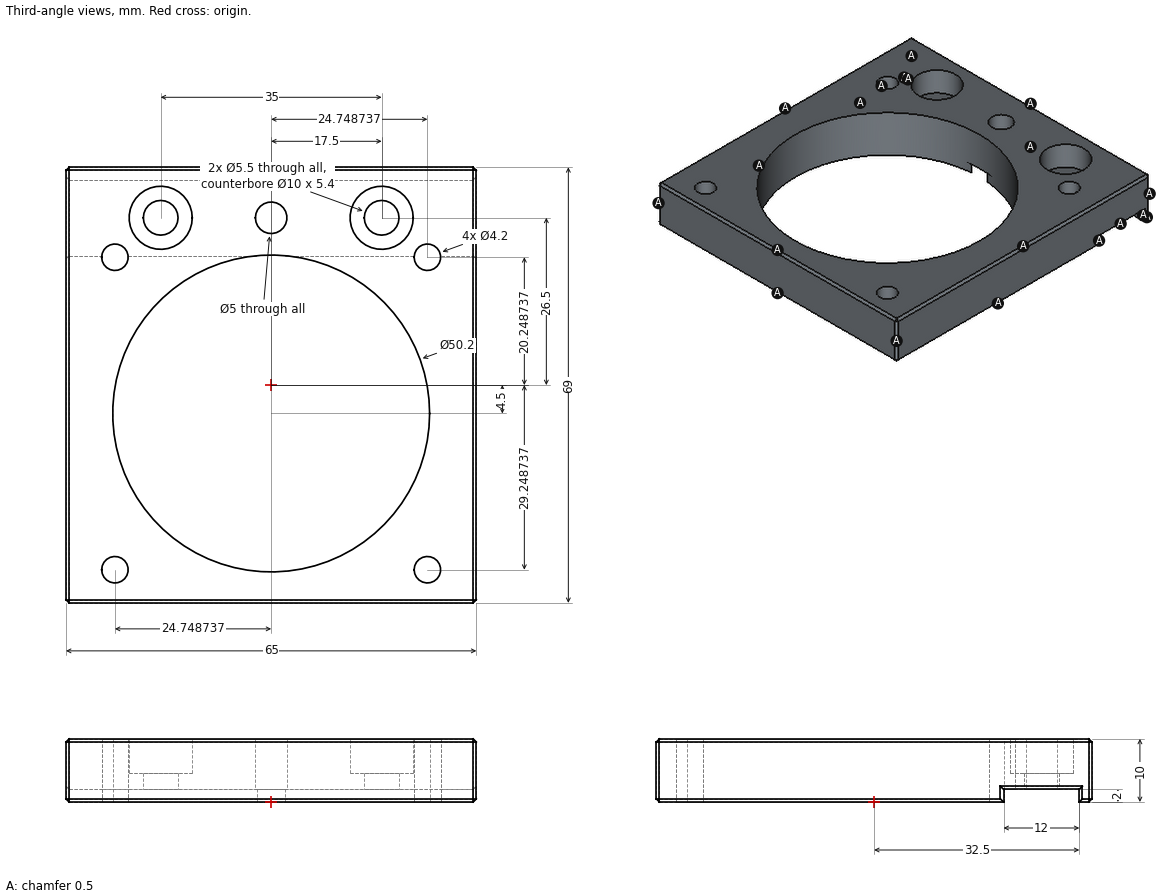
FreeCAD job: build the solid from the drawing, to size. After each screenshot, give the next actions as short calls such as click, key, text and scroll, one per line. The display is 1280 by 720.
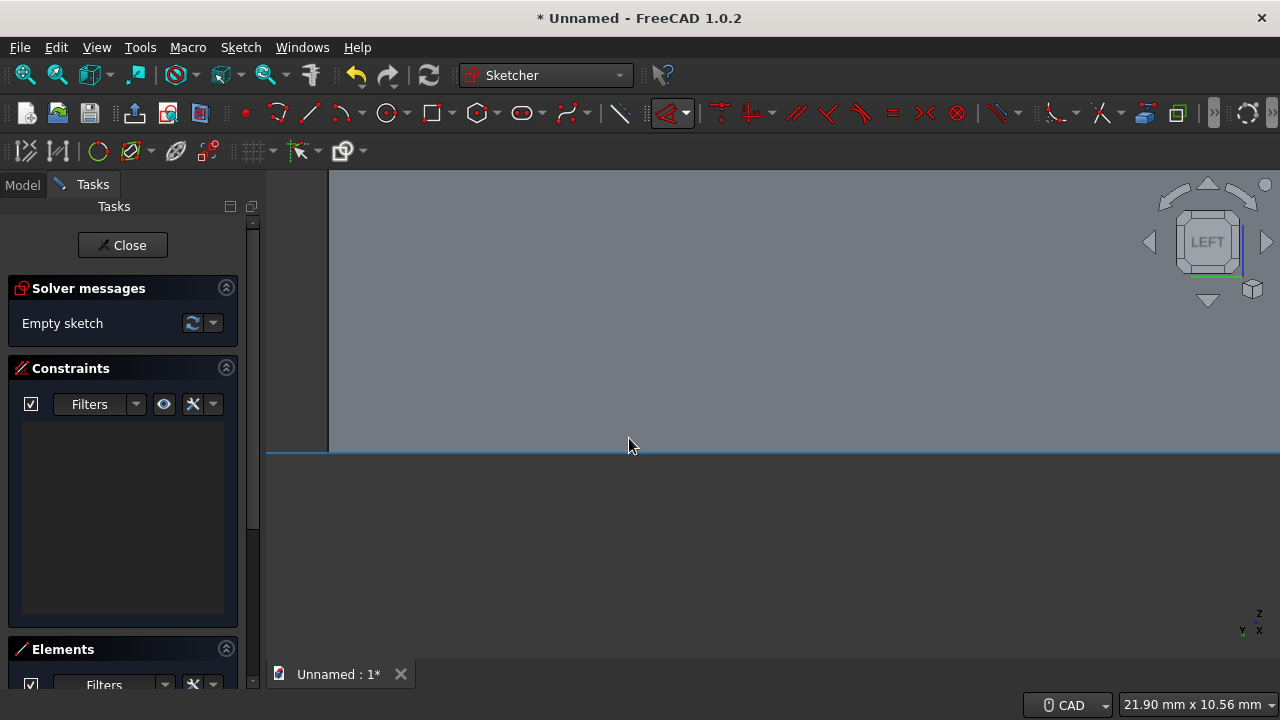
click(432, 114)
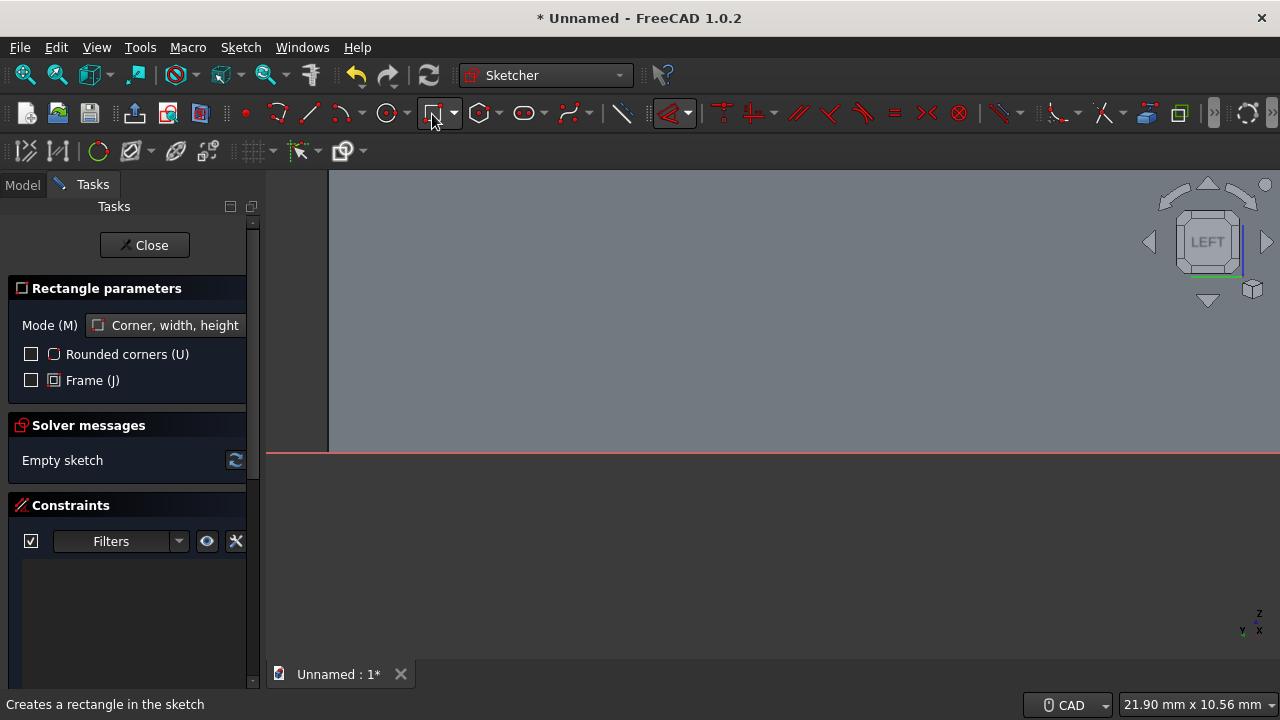
click(421, 360)
click(977, 453)
key(Escape)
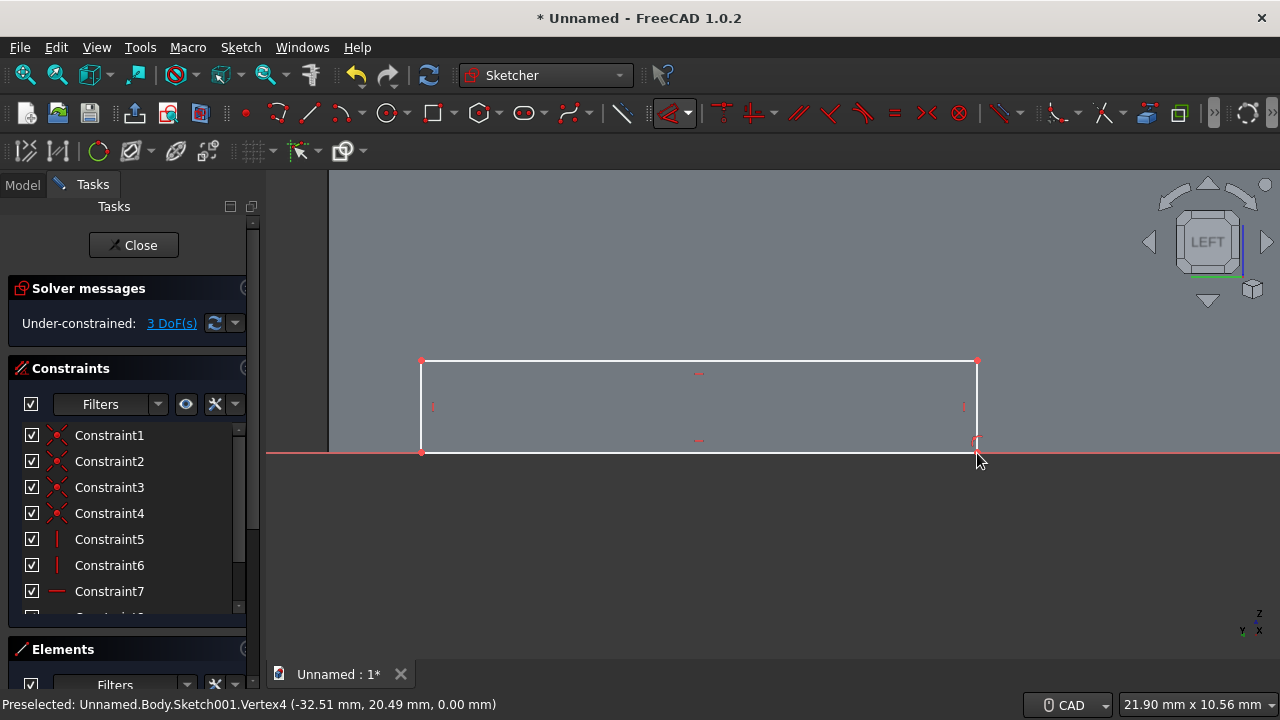
click(421, 389)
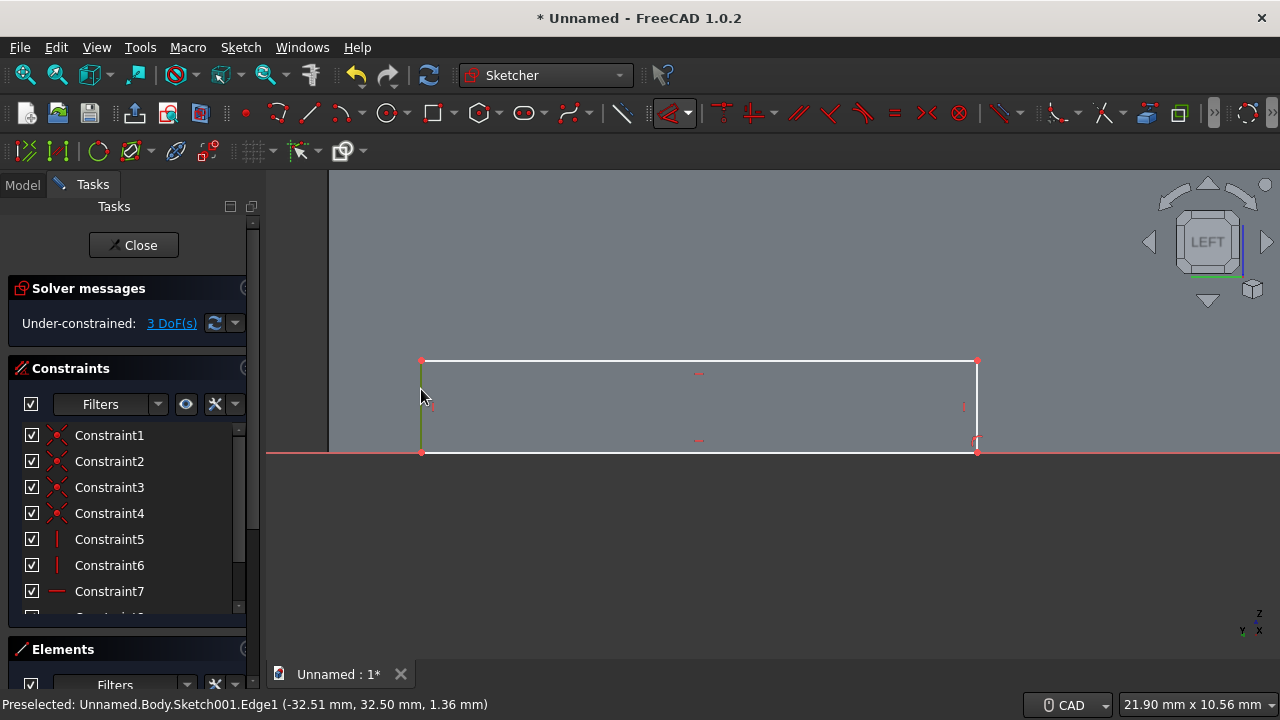
click(690, 114)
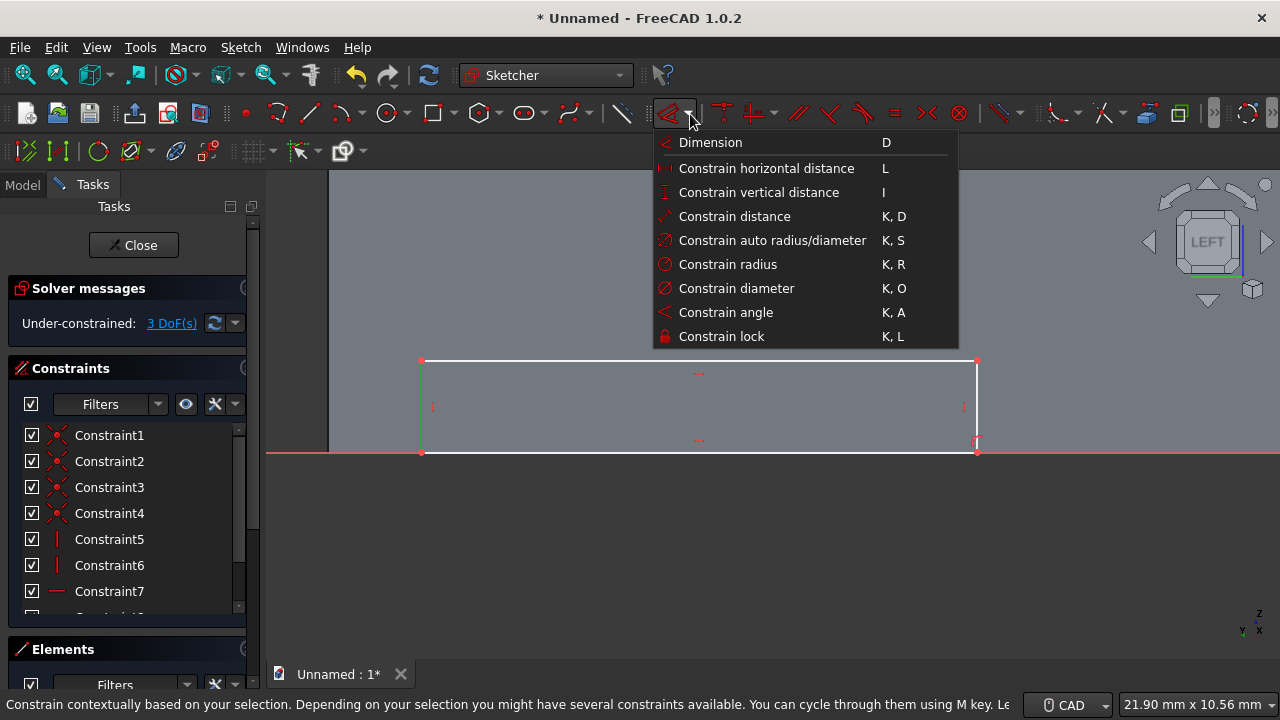
click(806, 192)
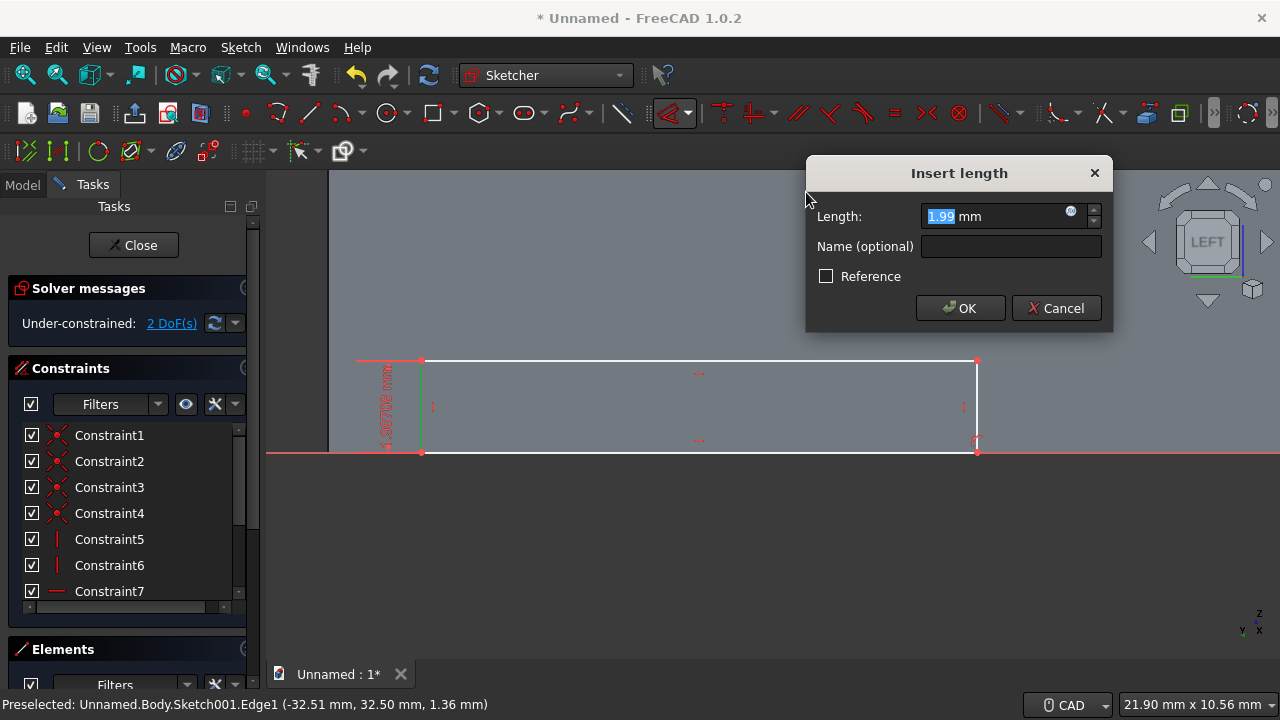
text(2)
key(Return)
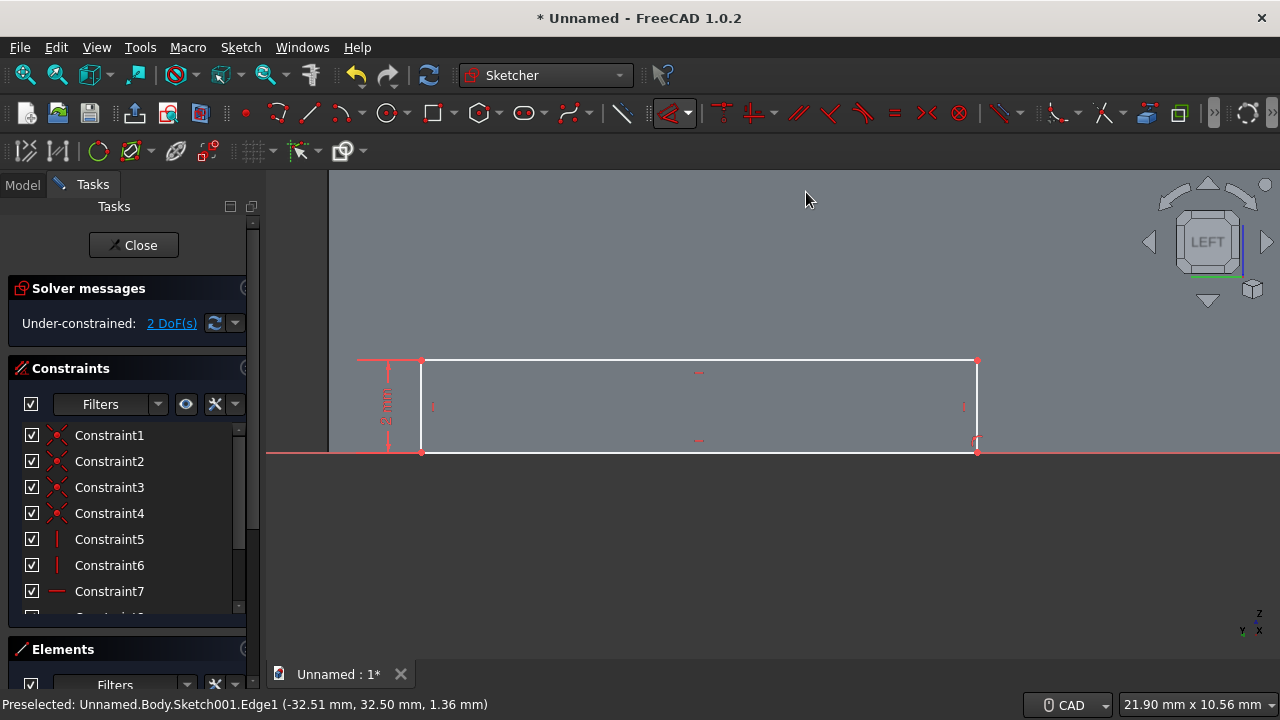
click(588, 453)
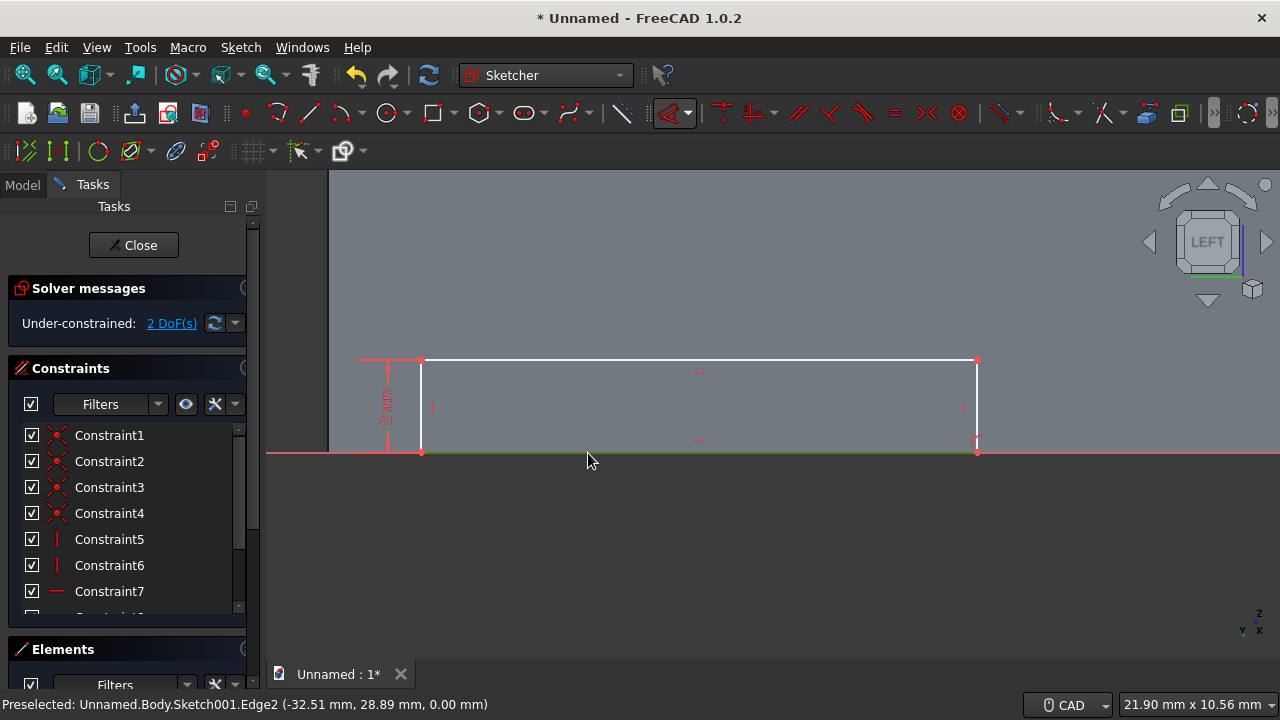
click(690, 114)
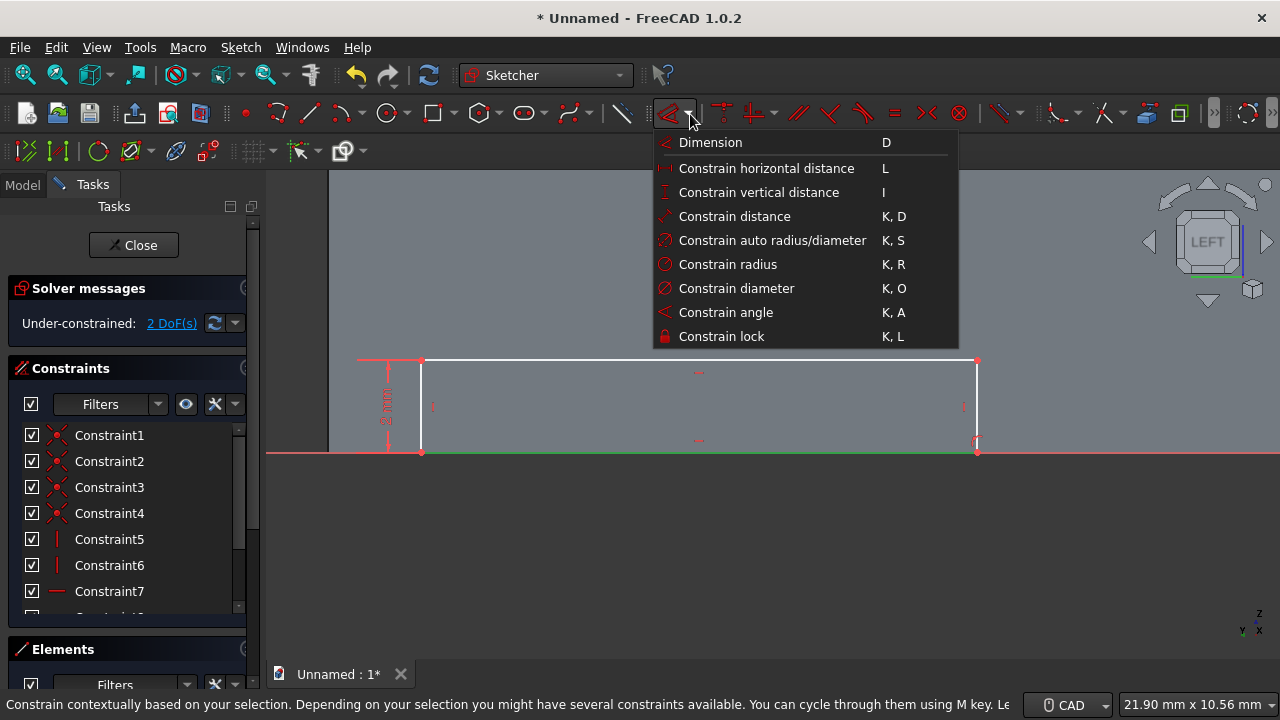
click(806, 168)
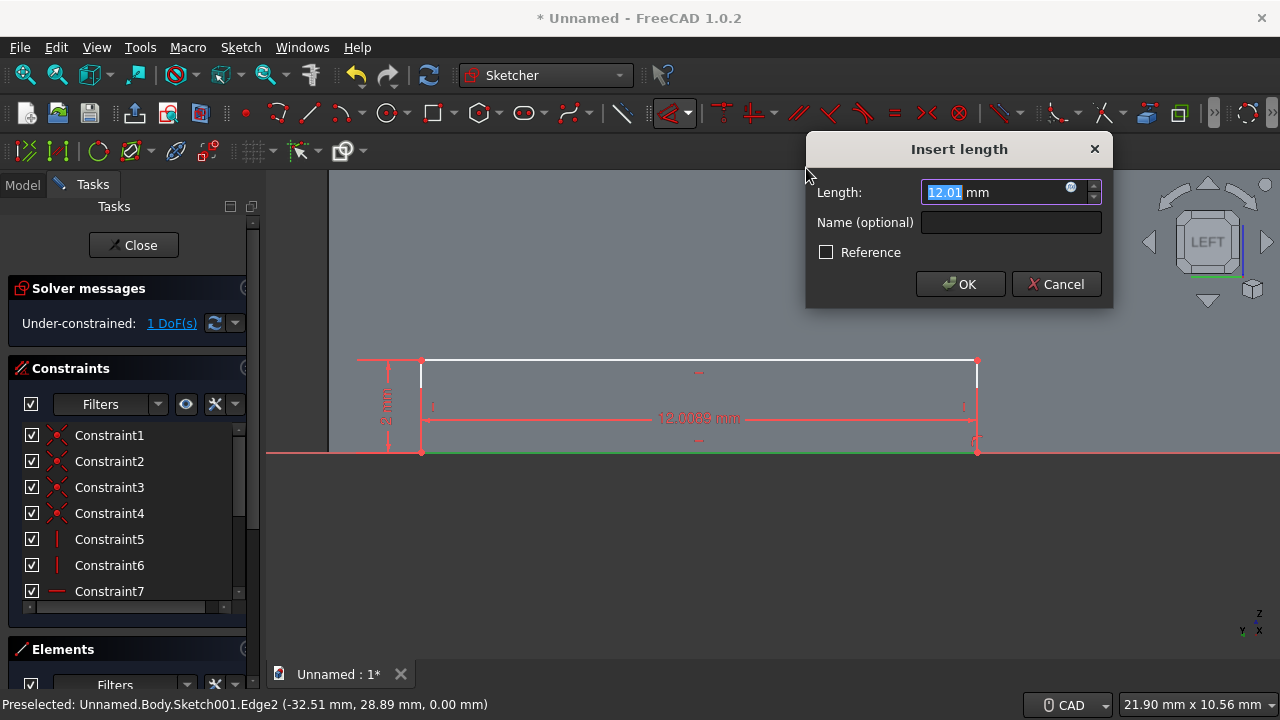
text(12)
key(Return)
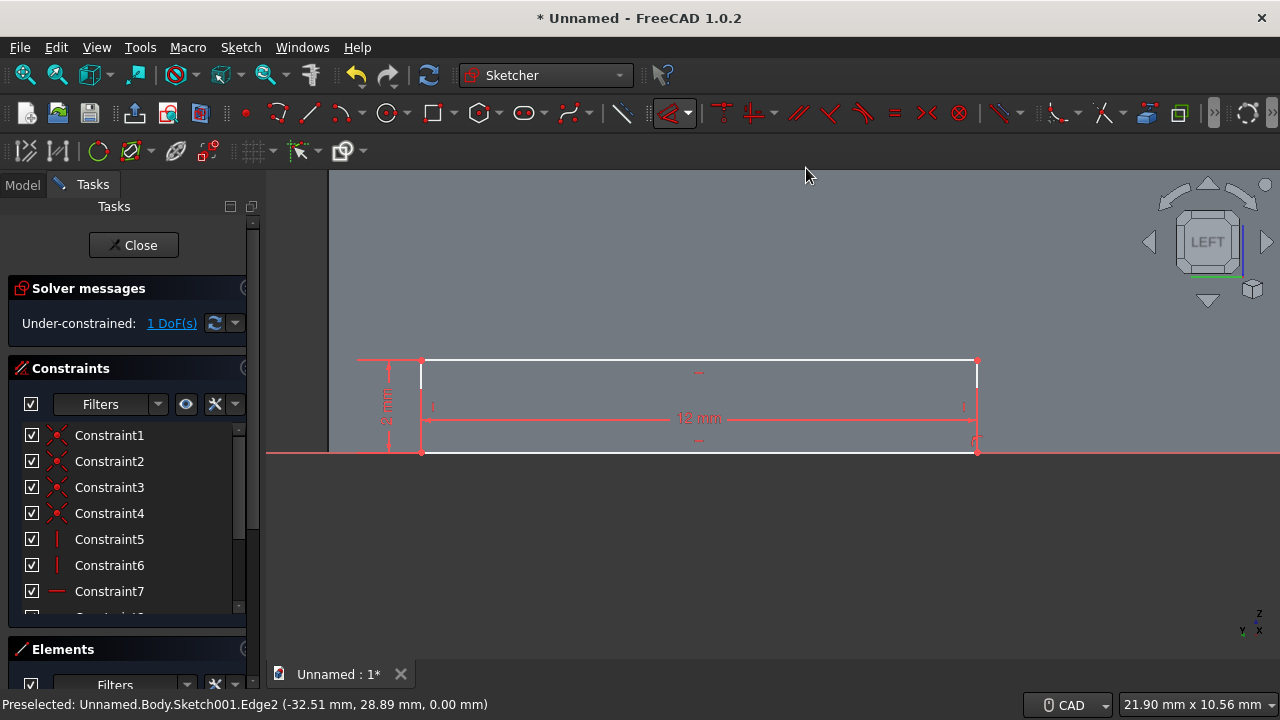
click(421, 360)